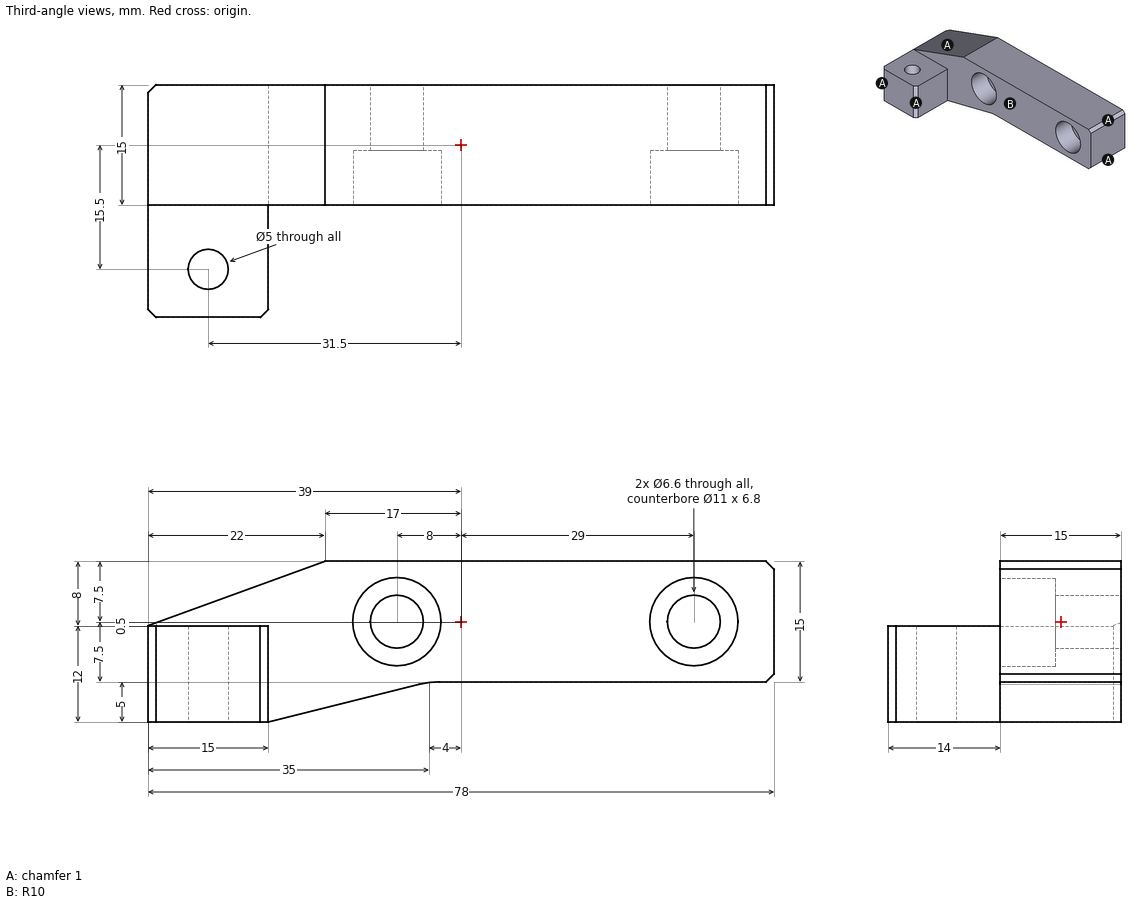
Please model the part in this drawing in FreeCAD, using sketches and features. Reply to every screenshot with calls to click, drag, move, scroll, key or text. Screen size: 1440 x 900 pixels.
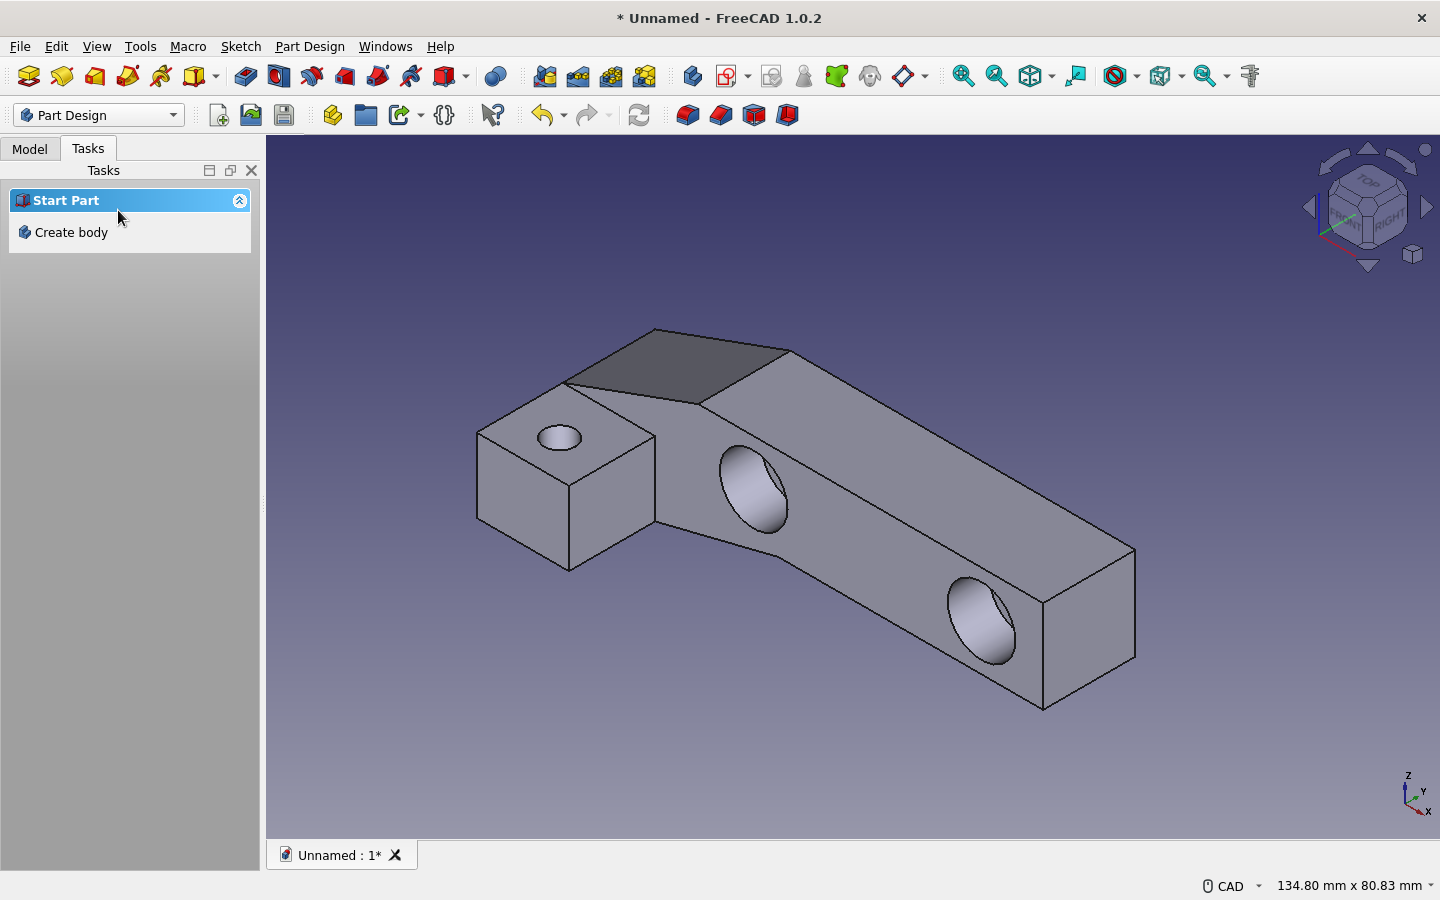
click(569, 528)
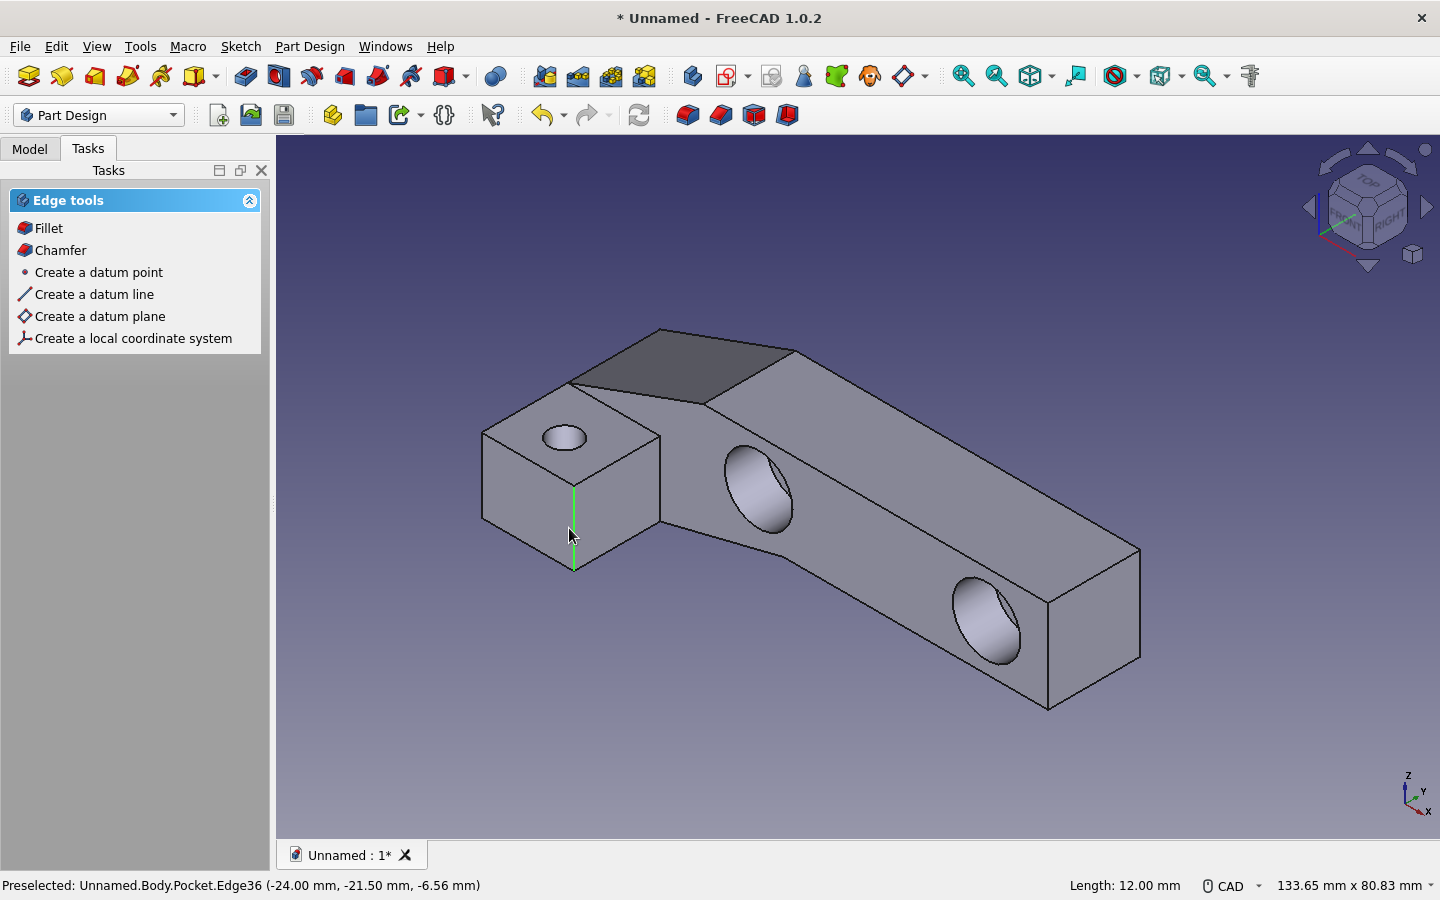
click(1094, 576, ctrl)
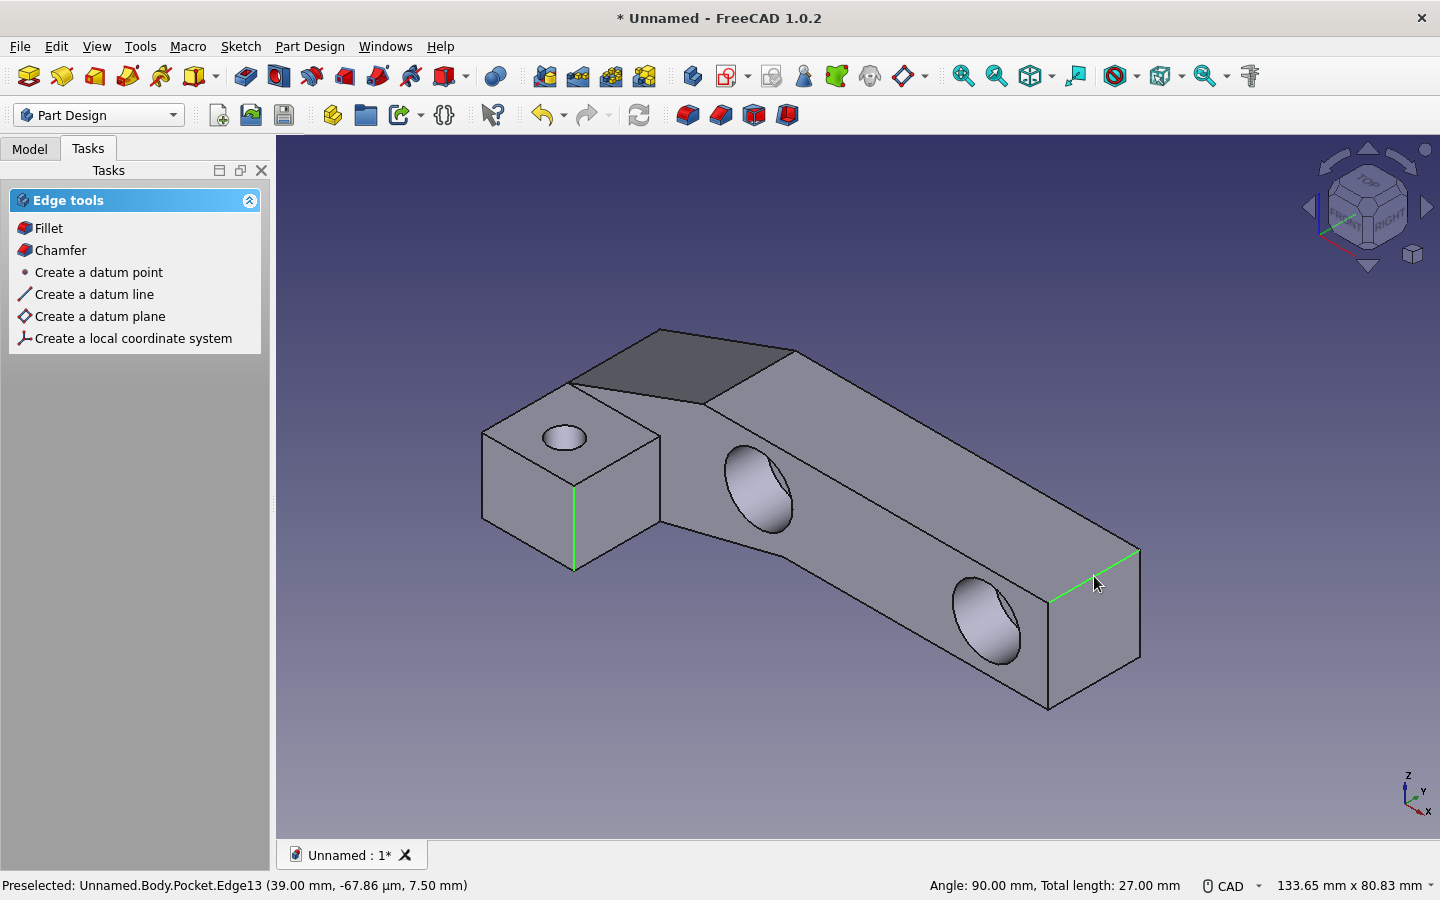
key(2)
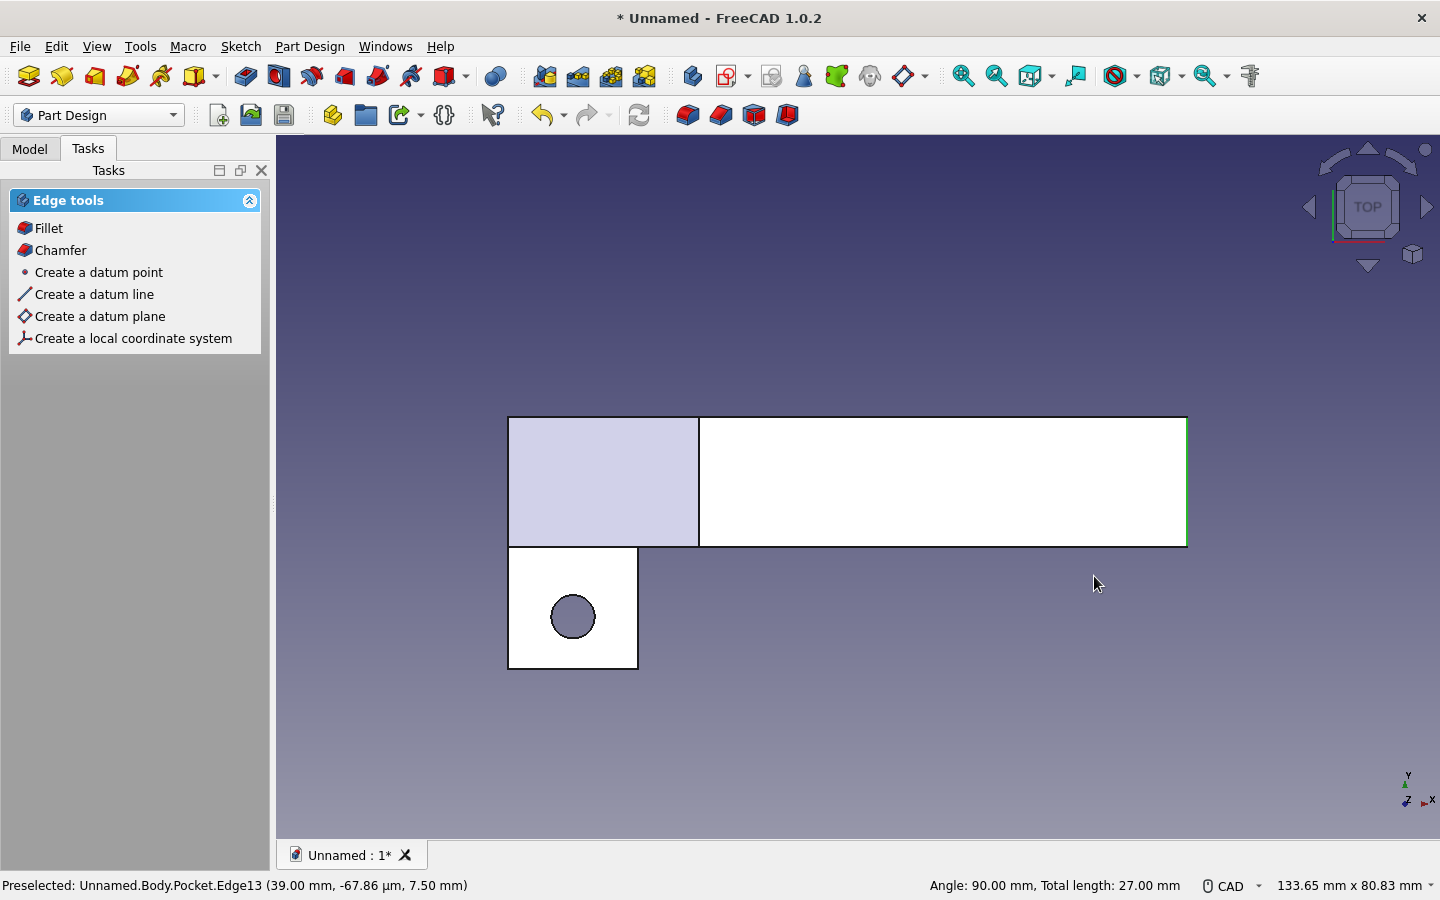
key(0)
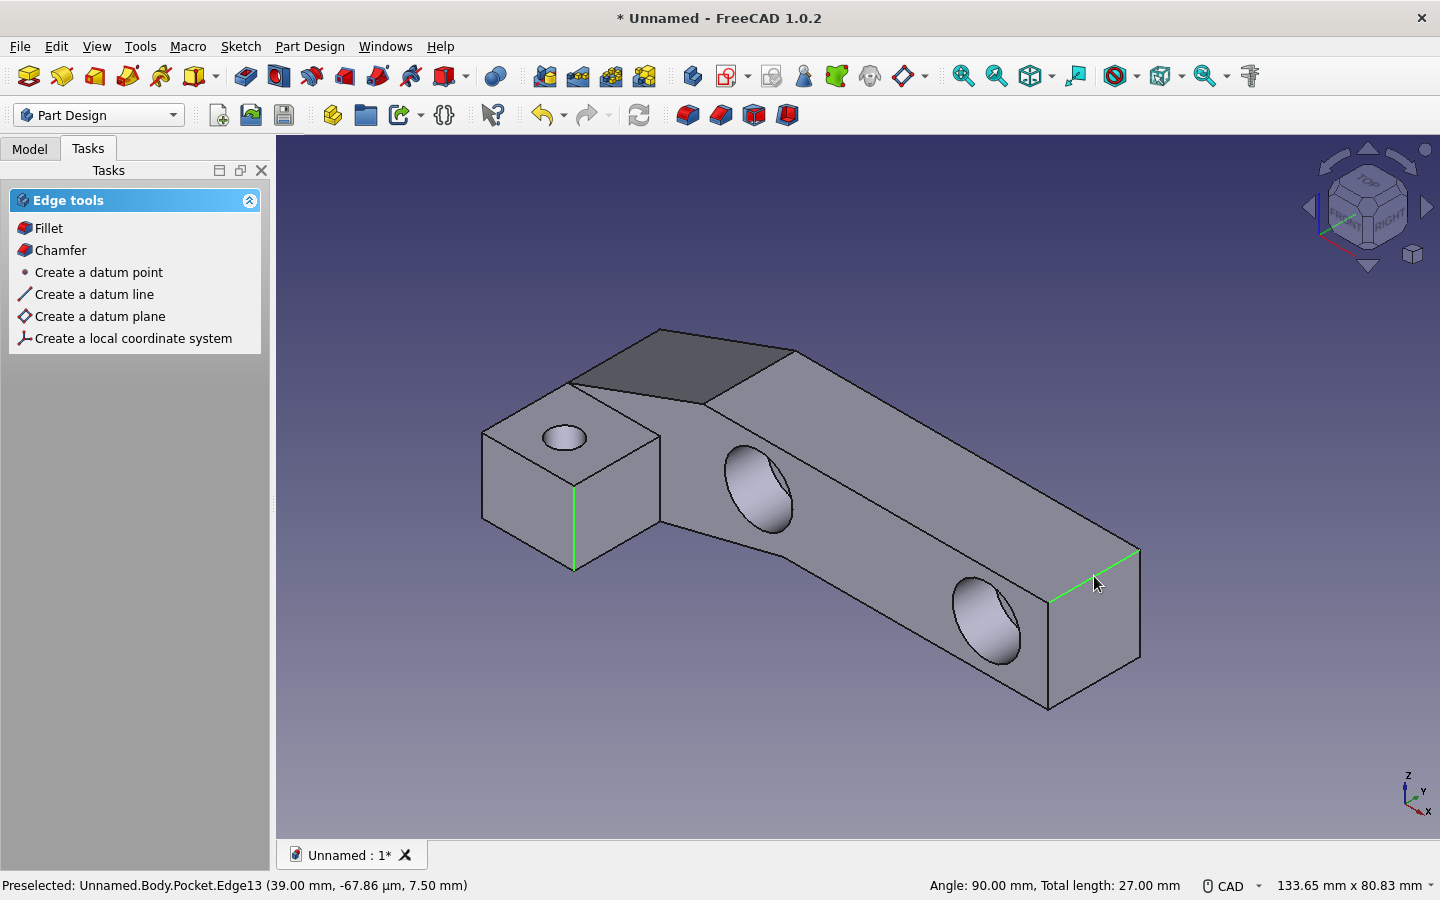
key(1)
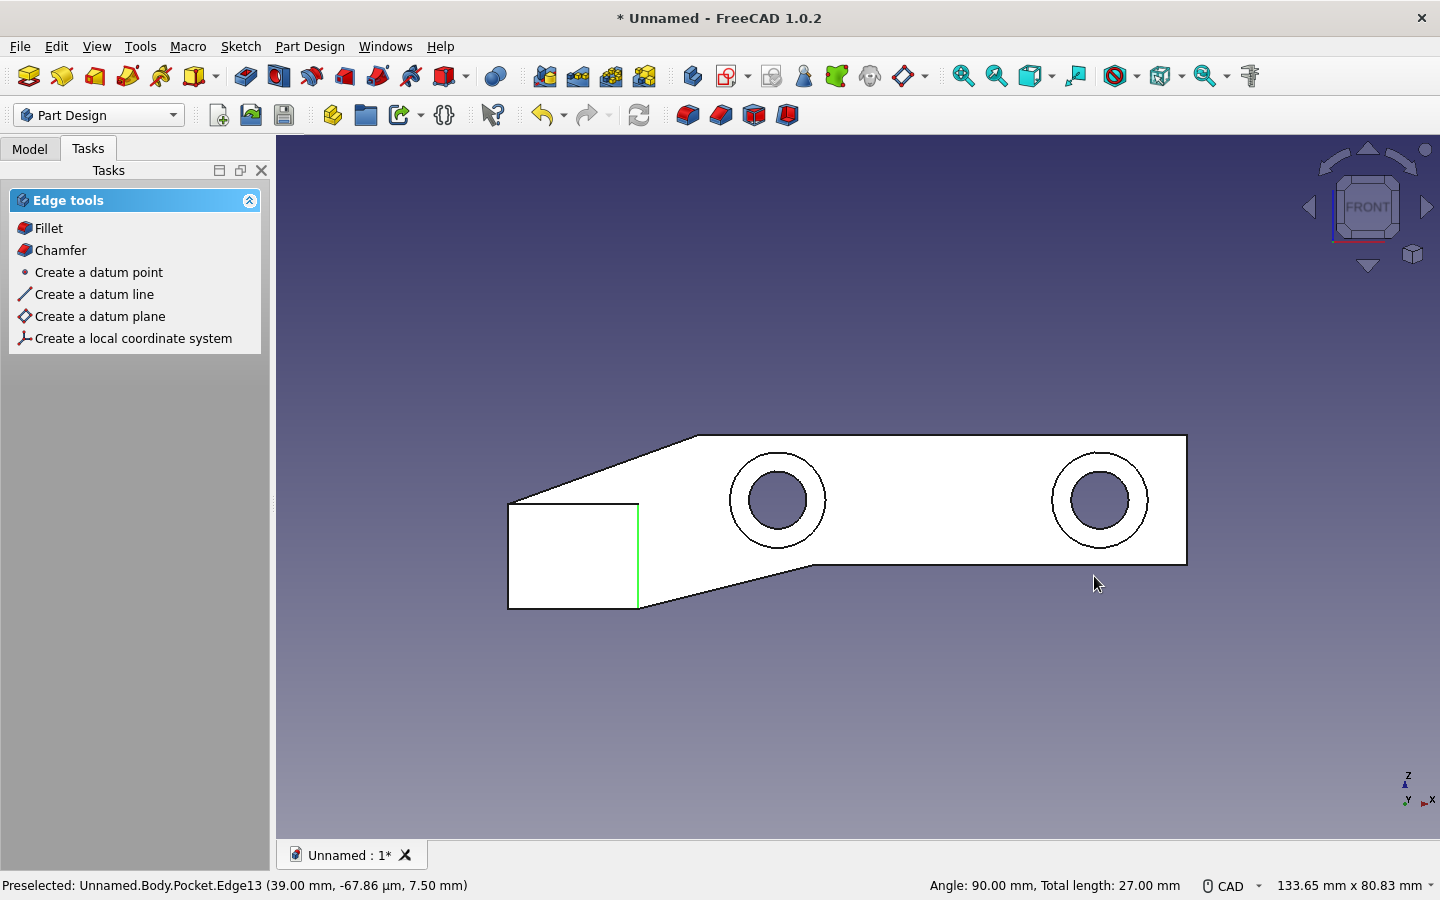
click(508, 556, ctrl)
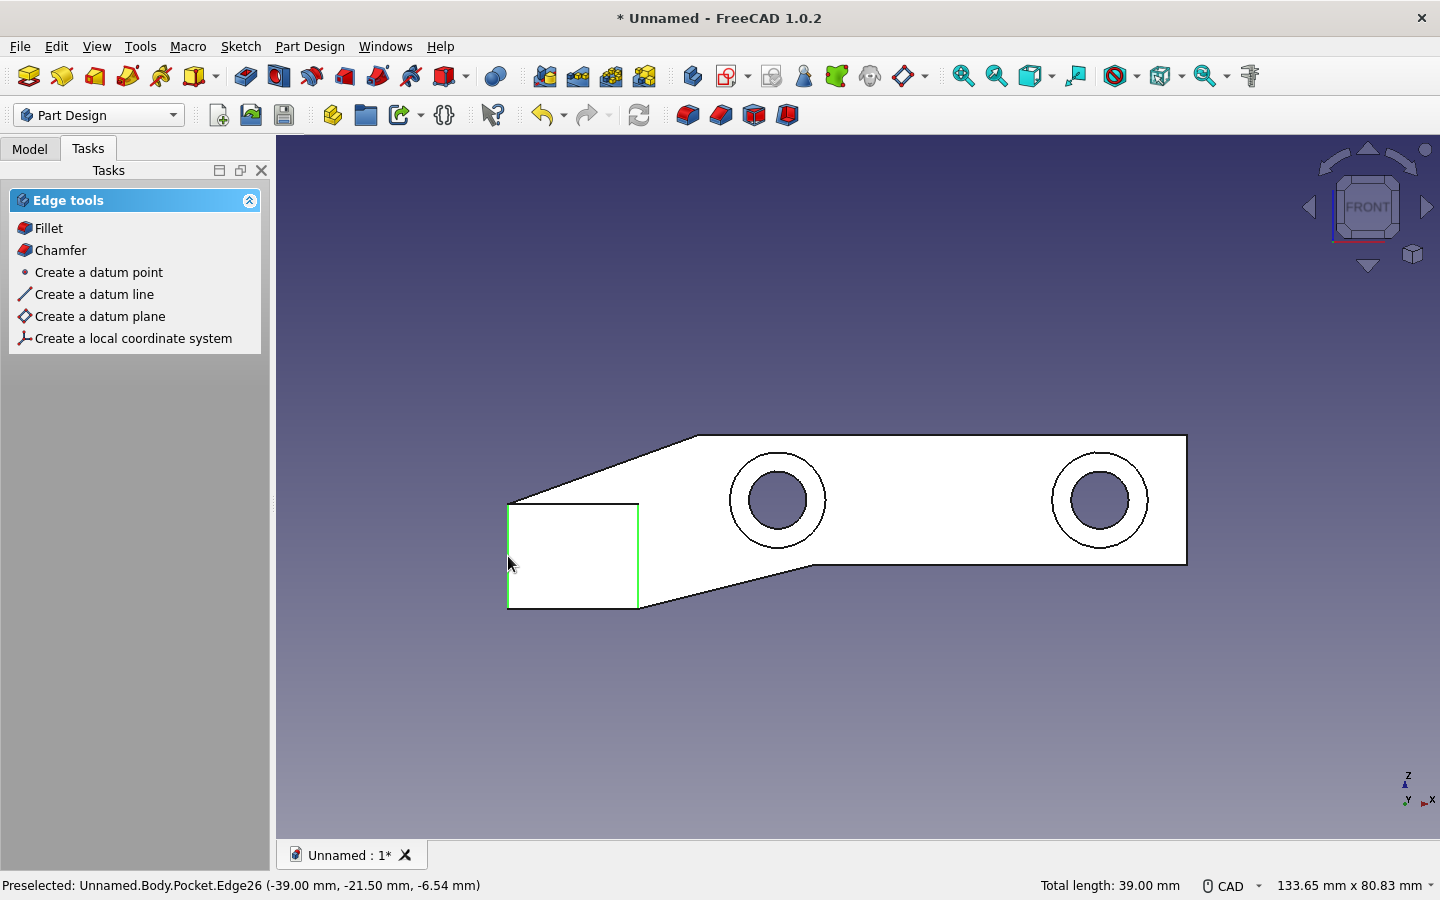
key(3)